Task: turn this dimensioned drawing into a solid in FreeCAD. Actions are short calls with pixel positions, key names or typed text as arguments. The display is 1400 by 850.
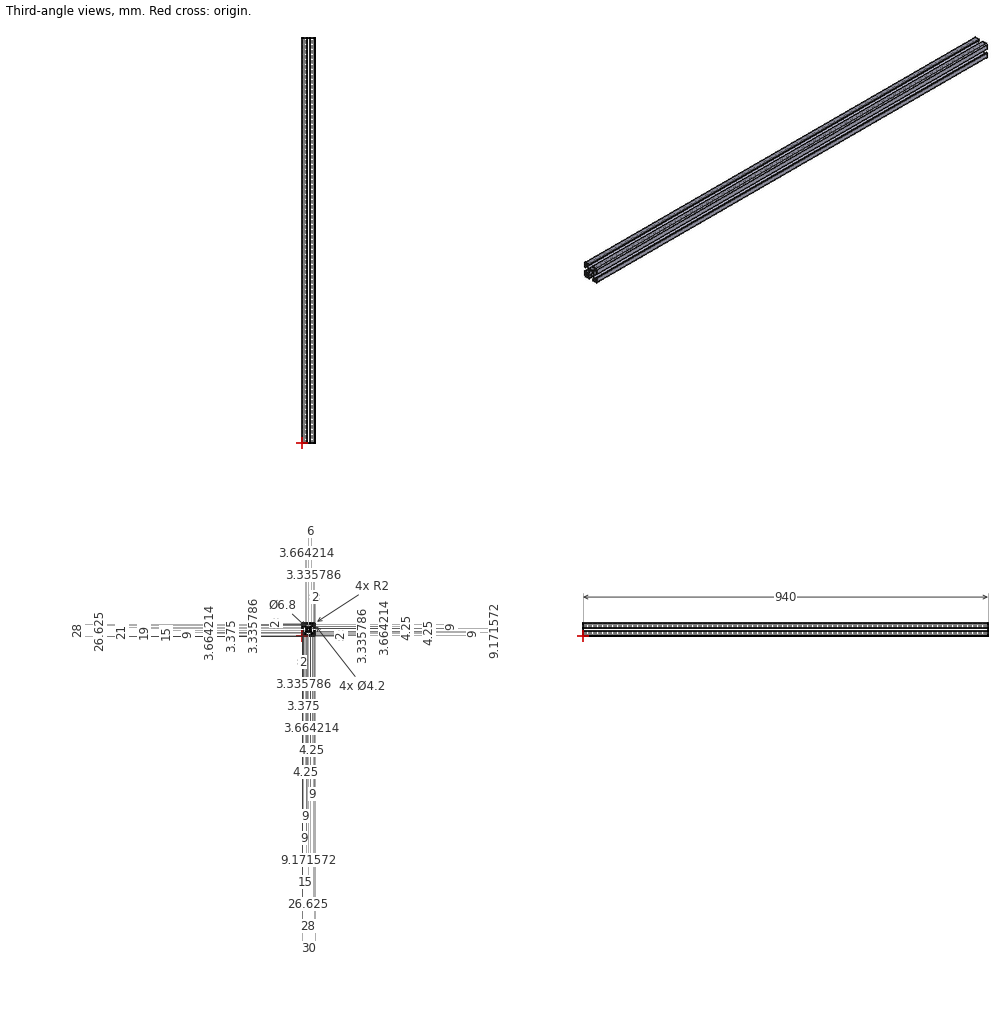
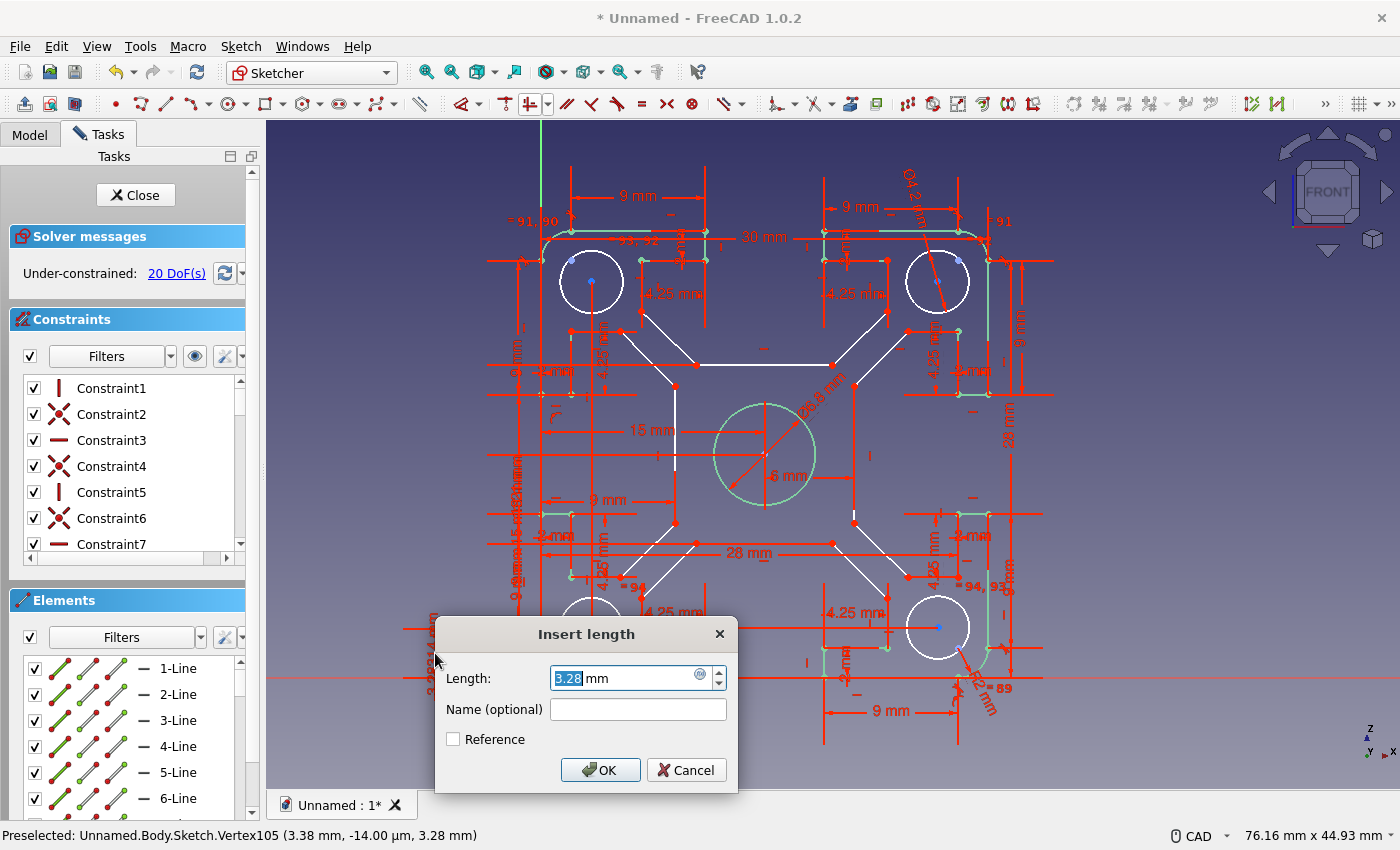
text(3.375)
key(Return)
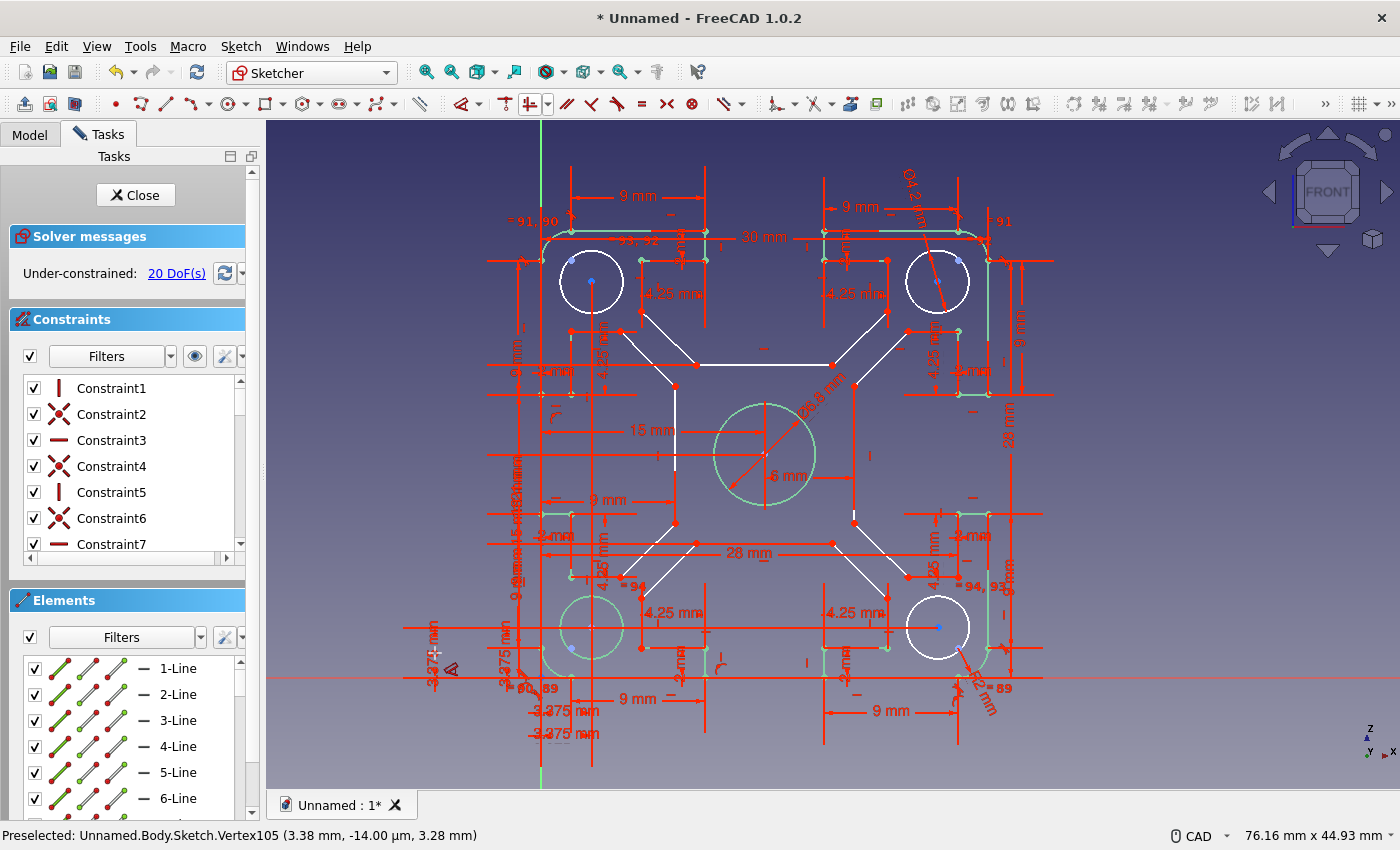
click(938, 282)
click(739, 712)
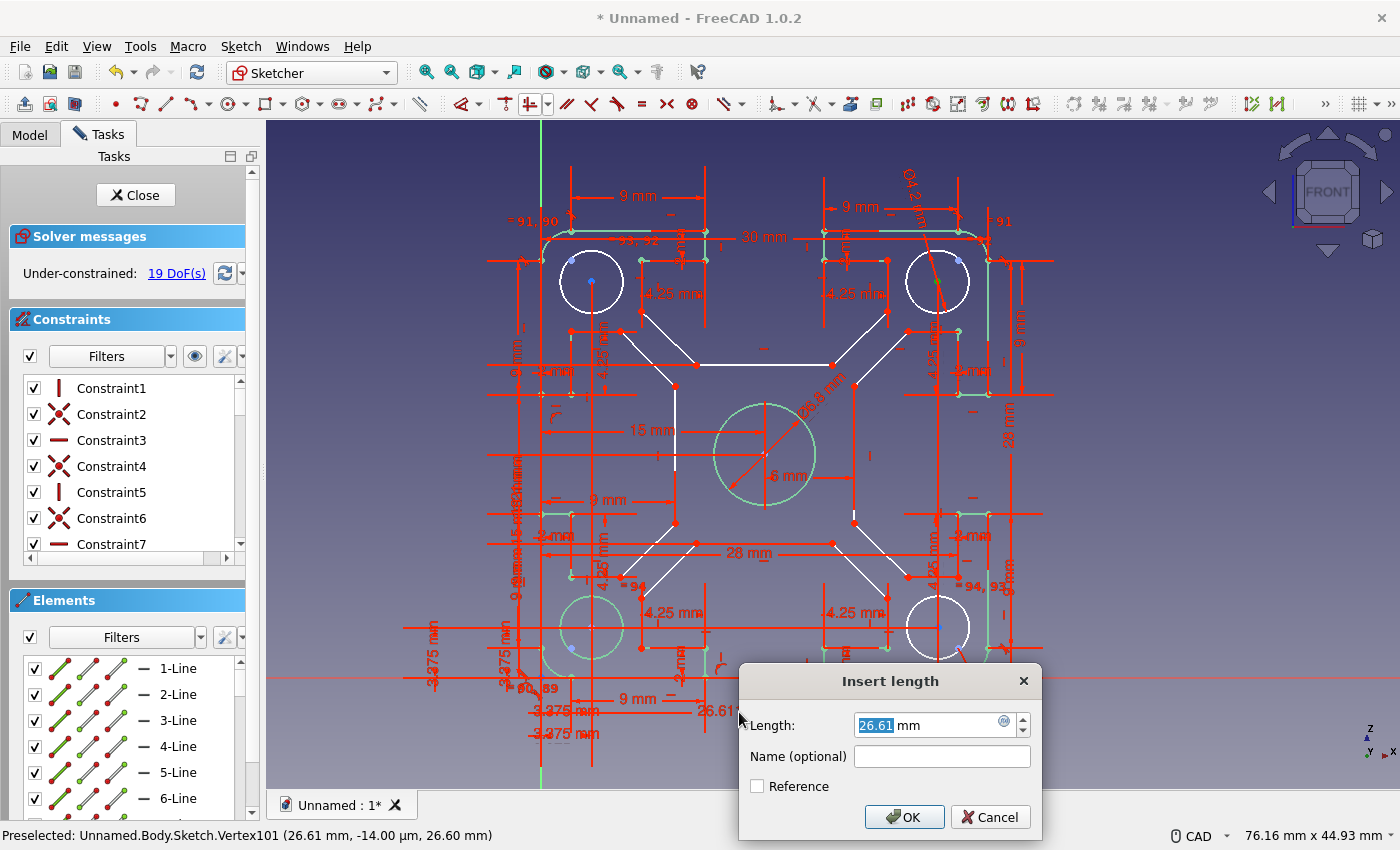
text(26.625)
key(Return)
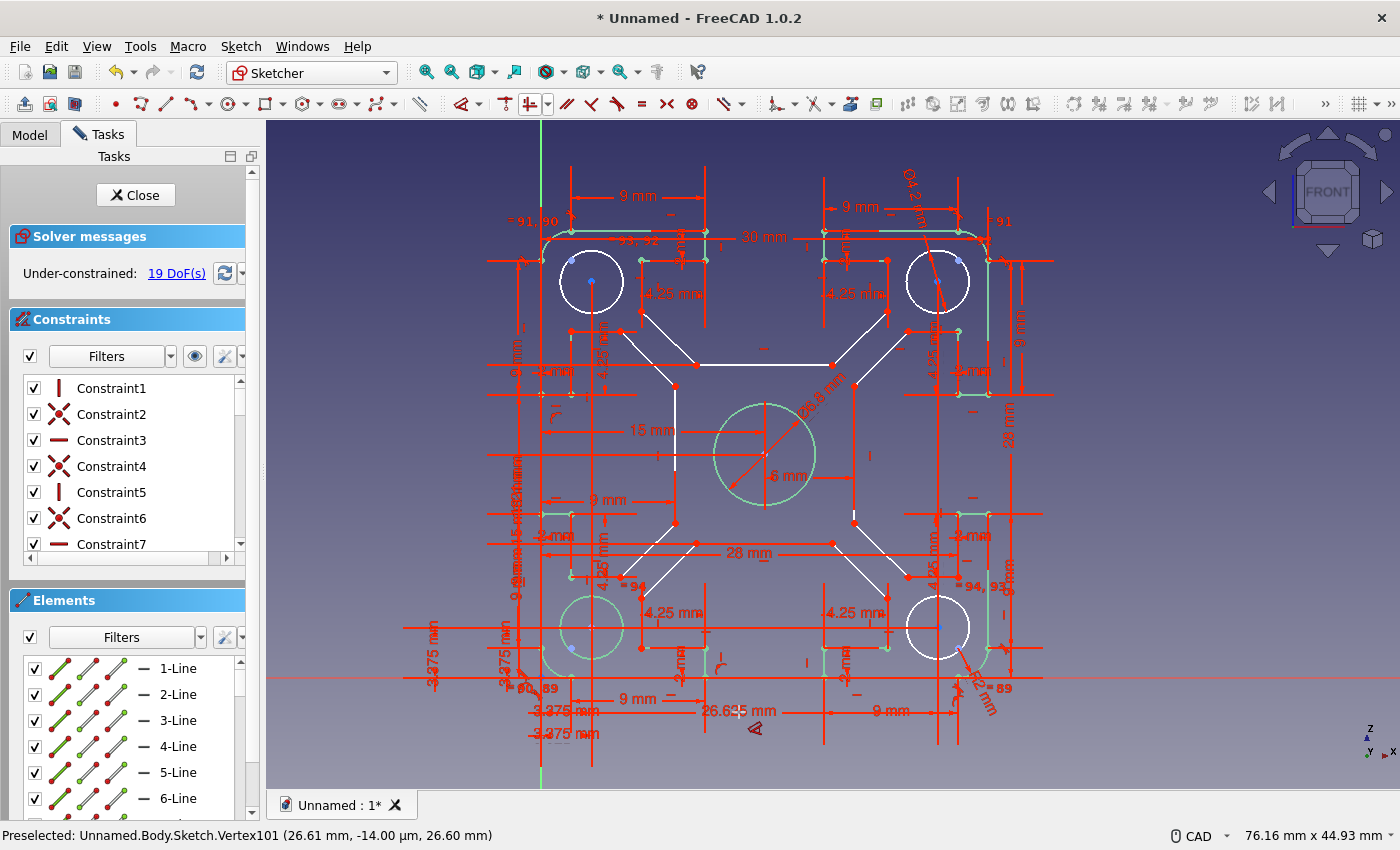
click(938, 282)
click(507, 618)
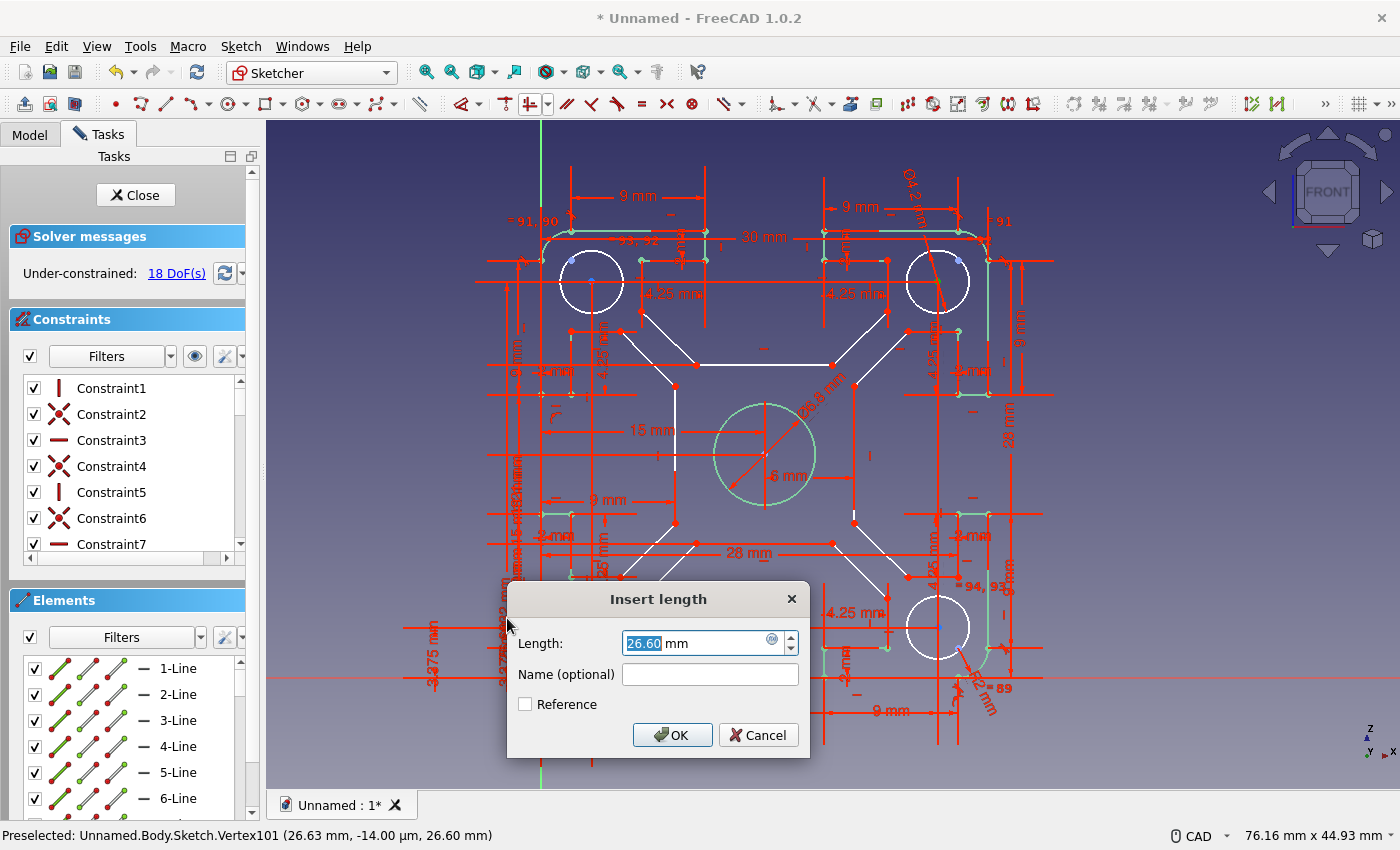
text(26.625)
key(Return)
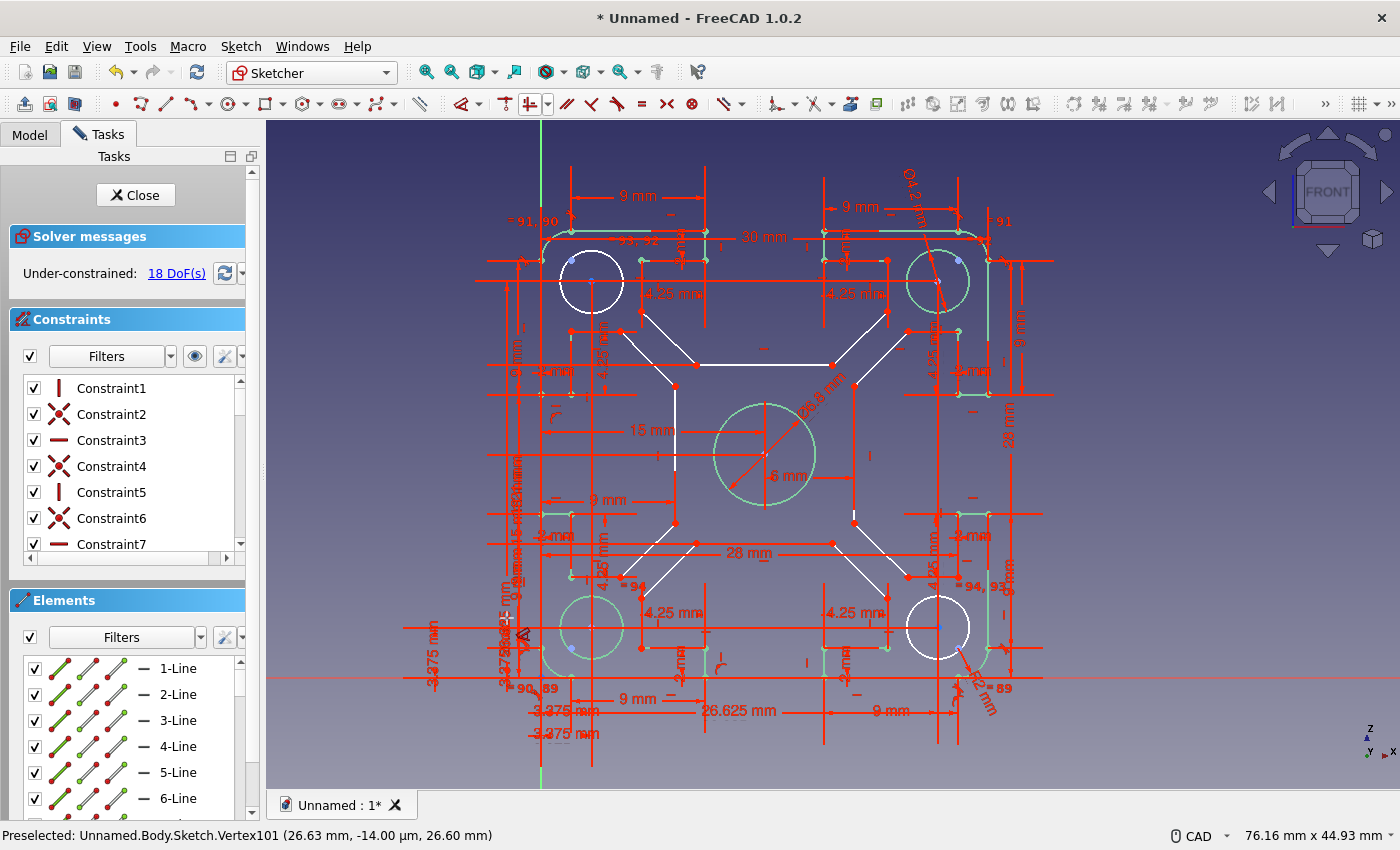
click(592, 282)
click(626, 480)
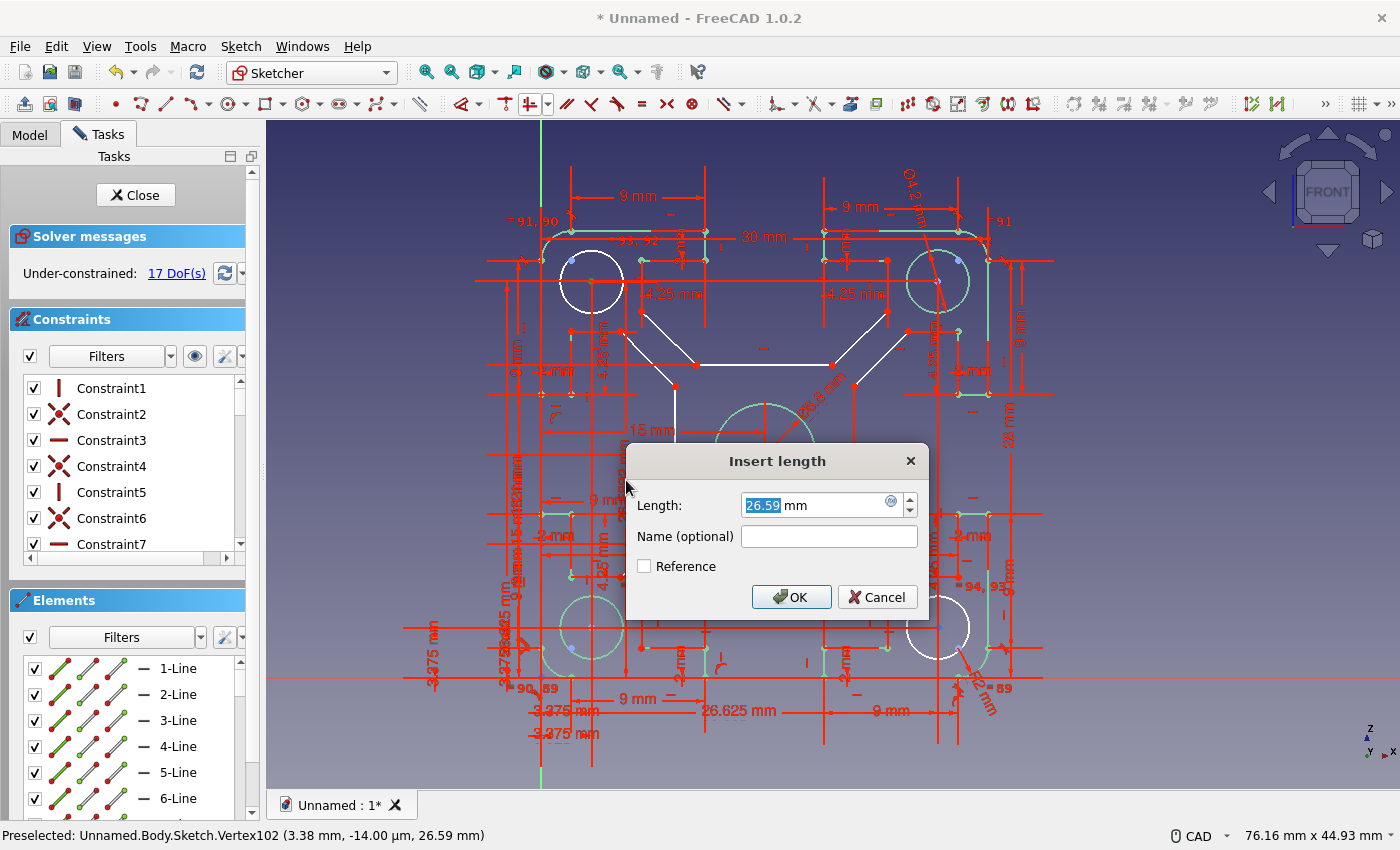
text(26.625)
key(Return)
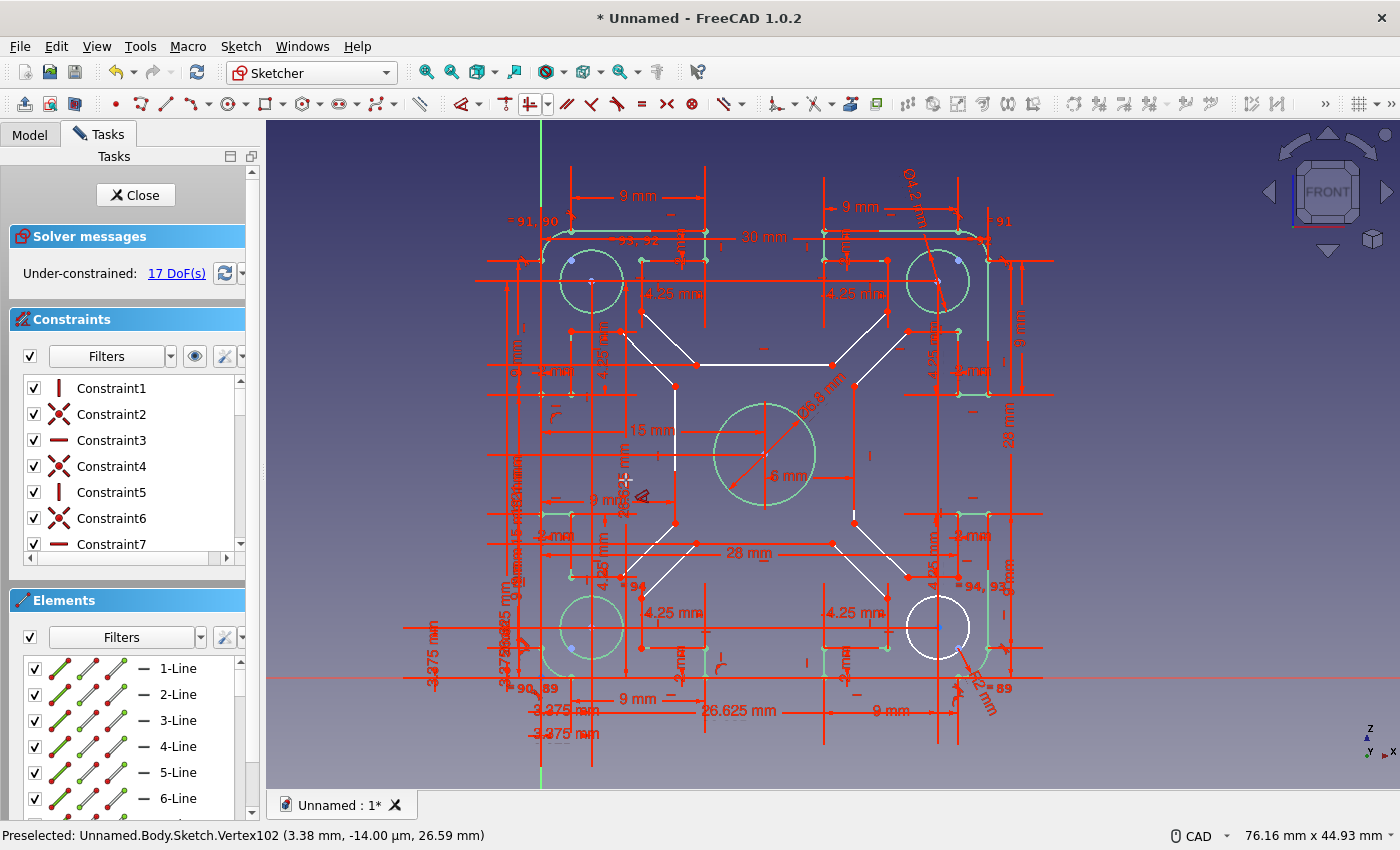
click(938, 628)
click(740, 594)